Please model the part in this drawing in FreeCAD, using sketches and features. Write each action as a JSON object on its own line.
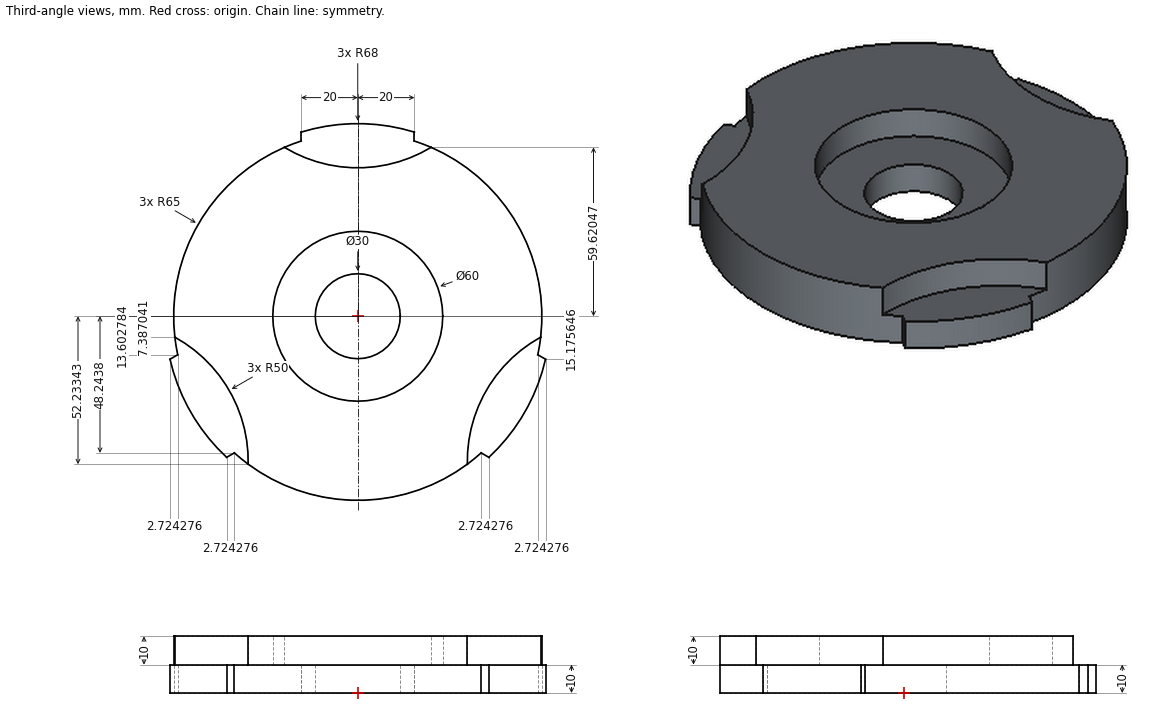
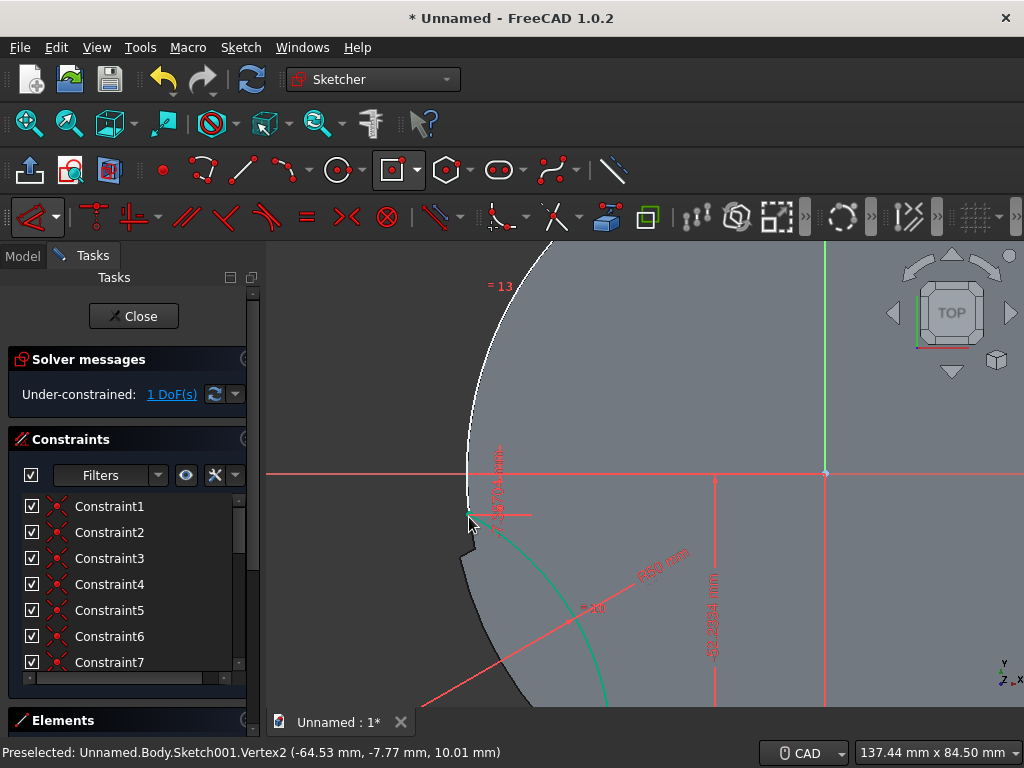
{"action": "scroll", "coordinate": [373, 462], "scroll_direction": "down", "scroll_amount": 4}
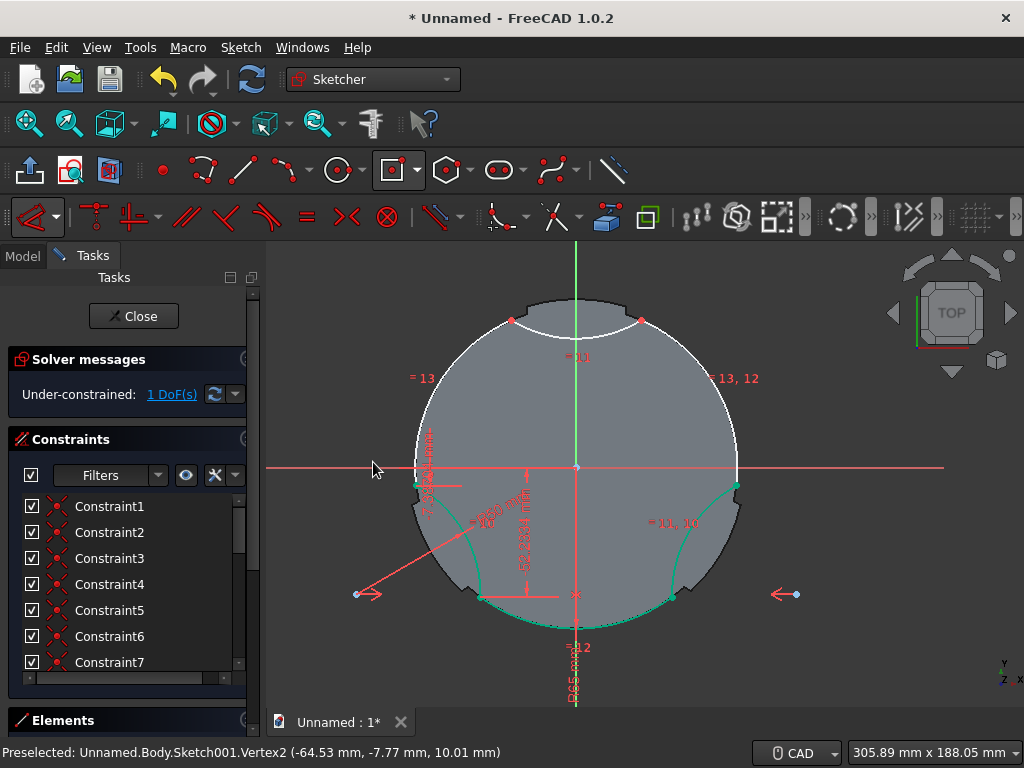
{"action": "left_click", "coordinate": [641, 320]}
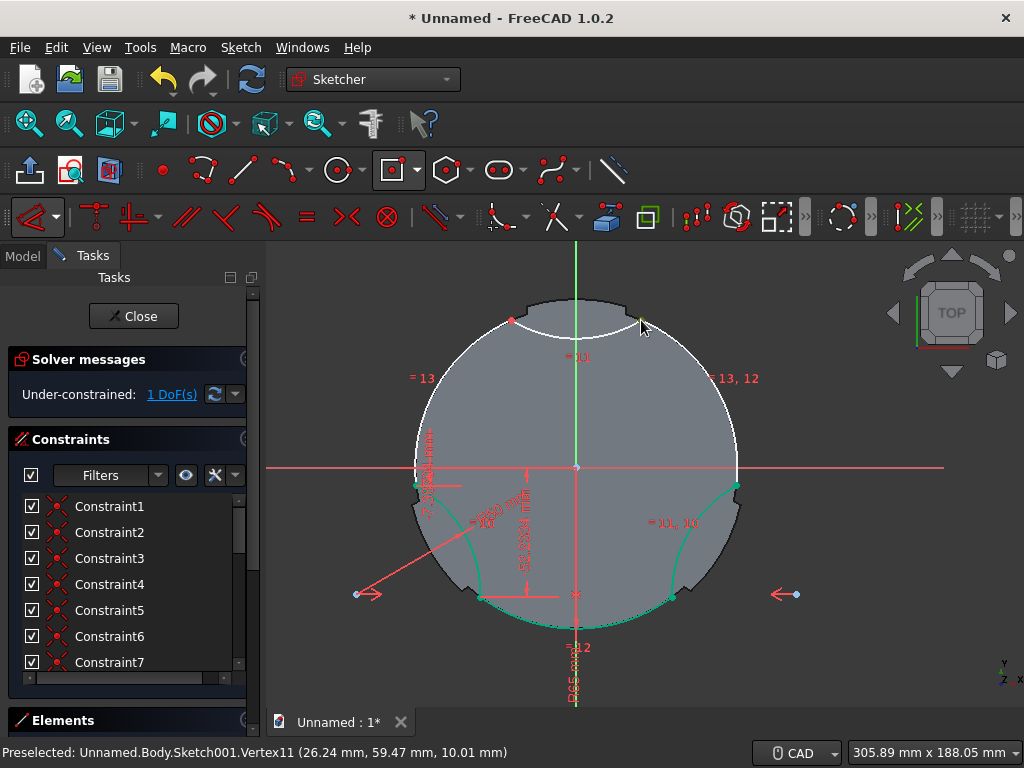
{"action": "left_click", "coordinate": [58, 218]}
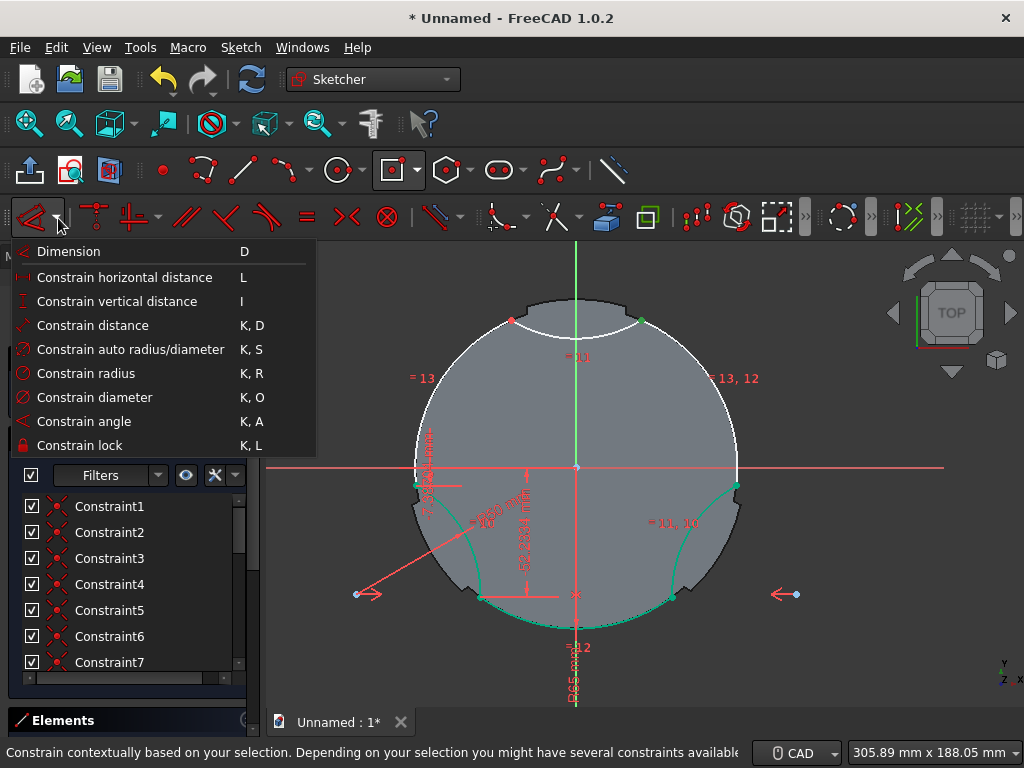
{"action": "left_click", "coordinate": [164, 301]}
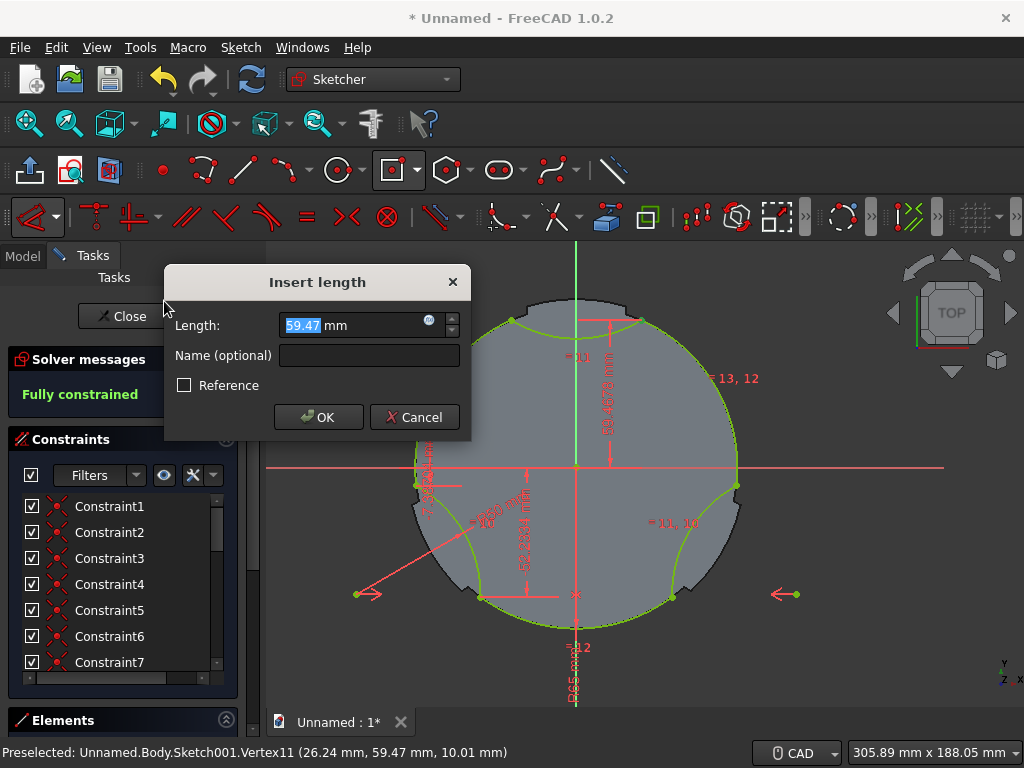
{"action": "type", "text": "59.62047"}
{"action": "key", "text": "Return"}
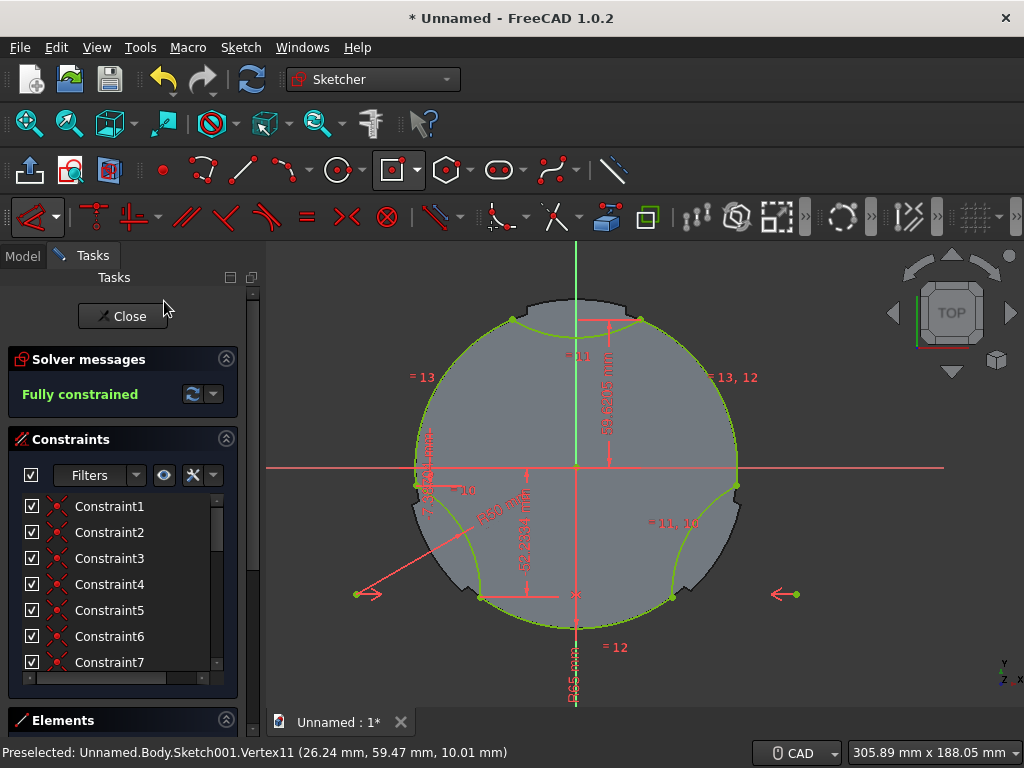
{"action": "left_click", "coordinate": [123, 316]}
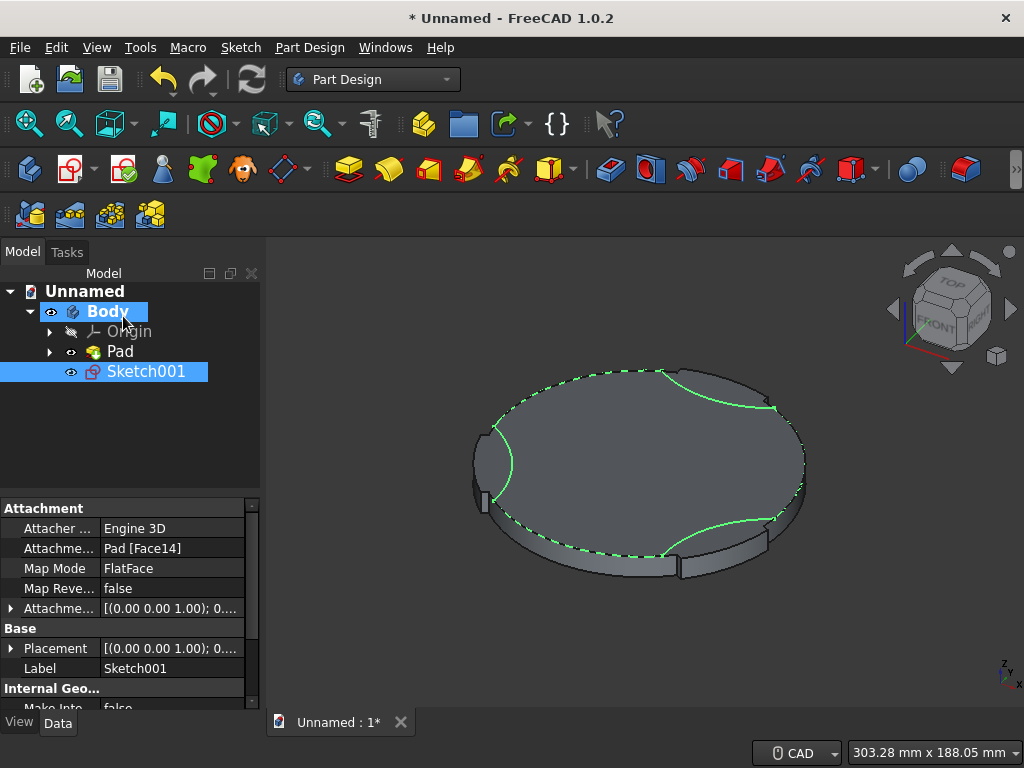
{"action": "left_click", "coordinate": [350, 170]}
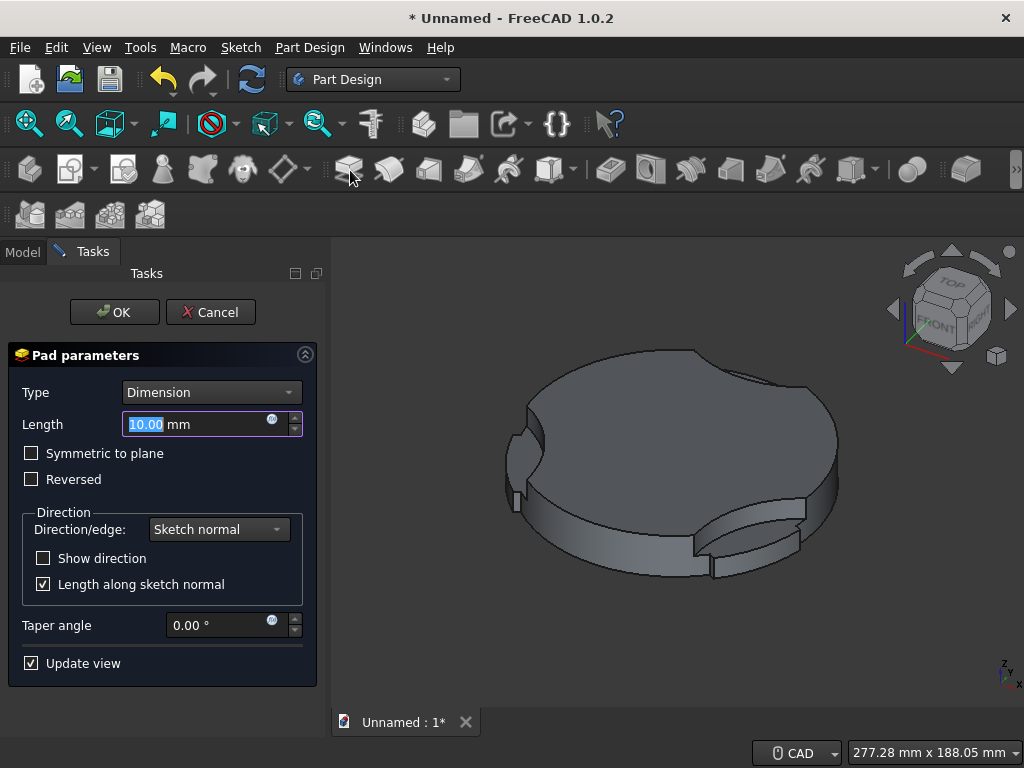
{"action": "type", "text": "10"}
{"action": "key", "text": "Tab"}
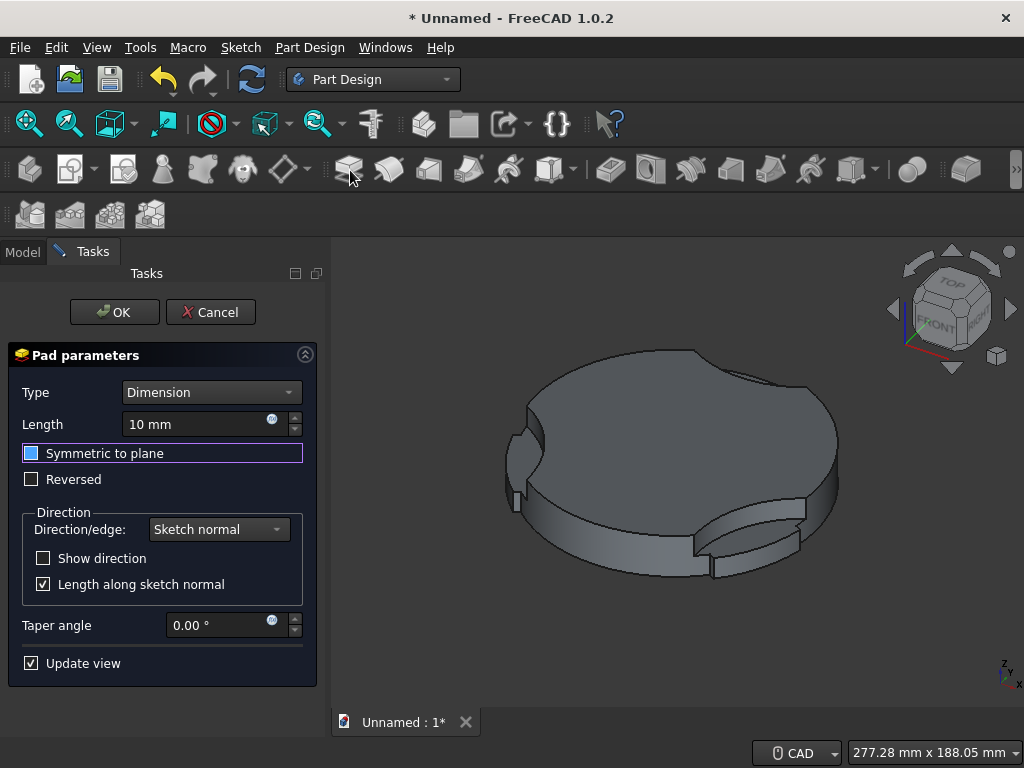
{"action": "left_click", "coordinate": [115, 312]}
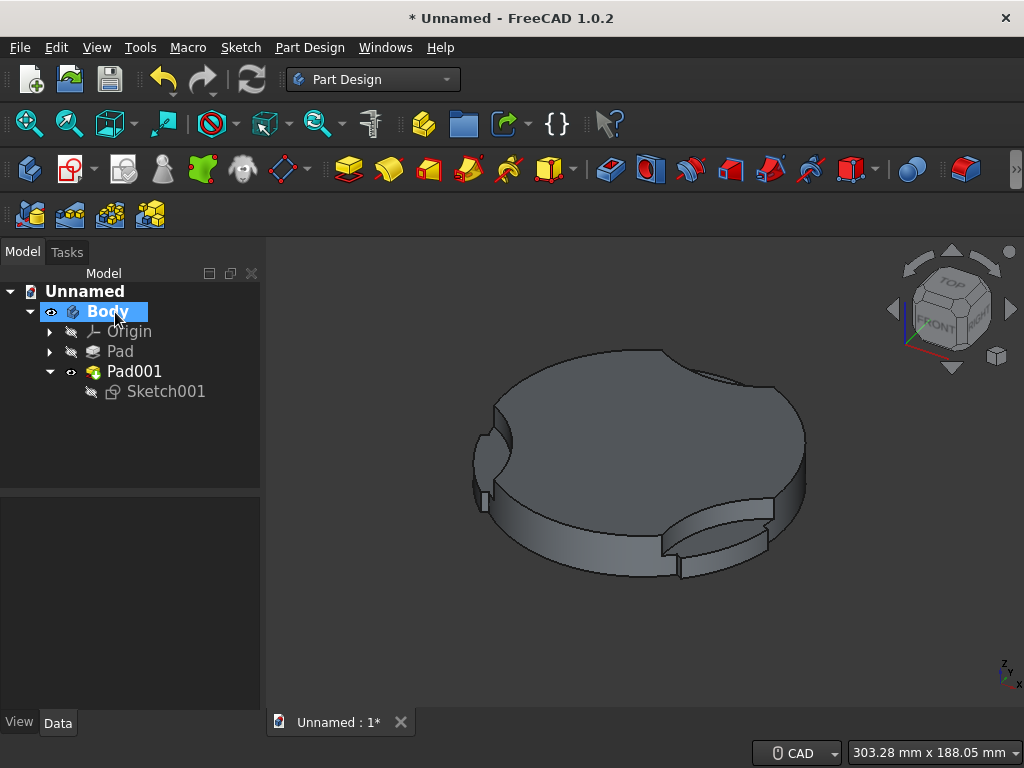
{"action": "left_click", "coordinate": [640, 445]}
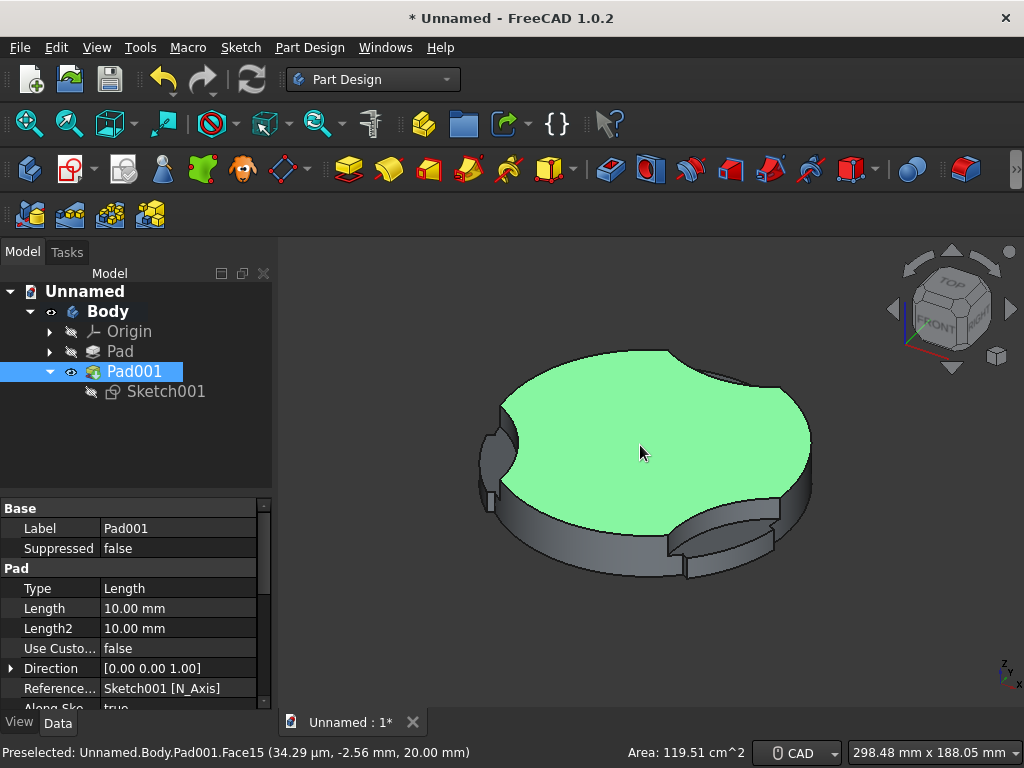
{"action": "left_click", "coordinate": [70, 170]}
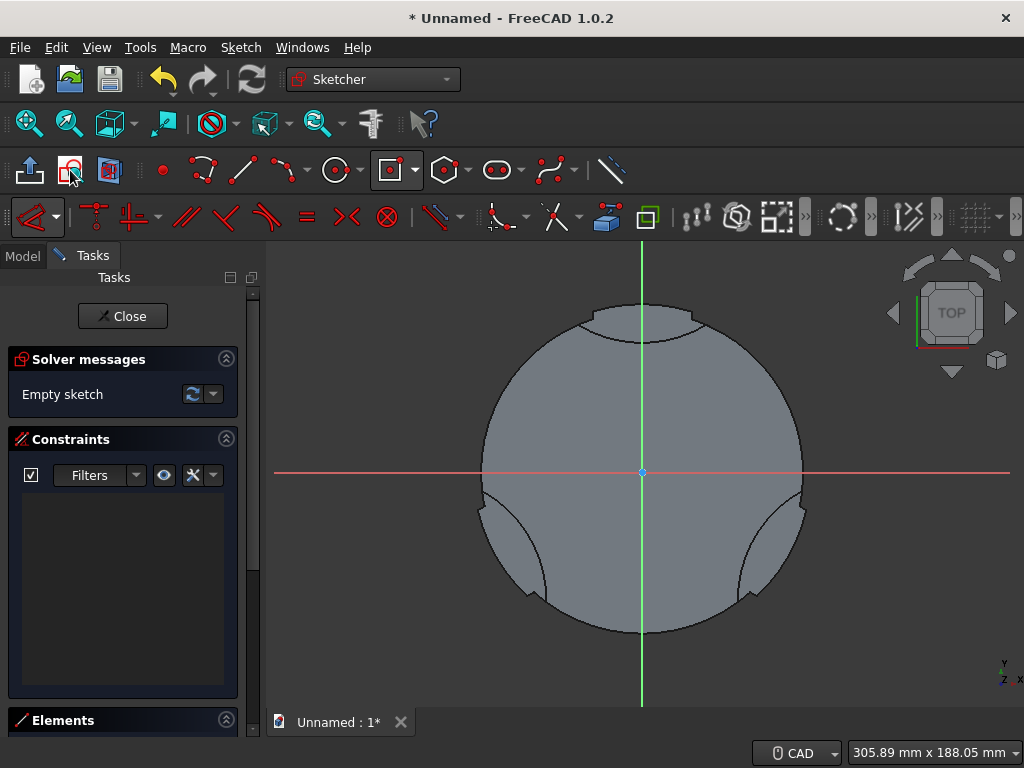
{"action": "scroll", "coordinate": [722, 471], "scroll_direction": "up", "scroll_amount": 3}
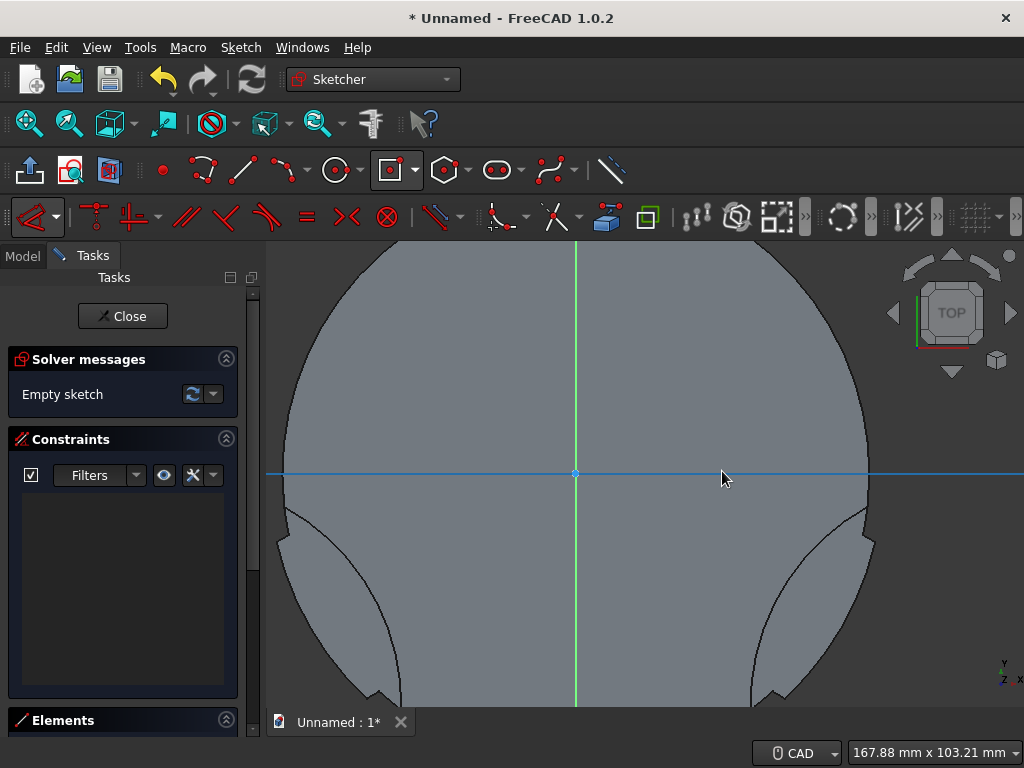
{"action": "left_click", "coordinate": [336, 170]}